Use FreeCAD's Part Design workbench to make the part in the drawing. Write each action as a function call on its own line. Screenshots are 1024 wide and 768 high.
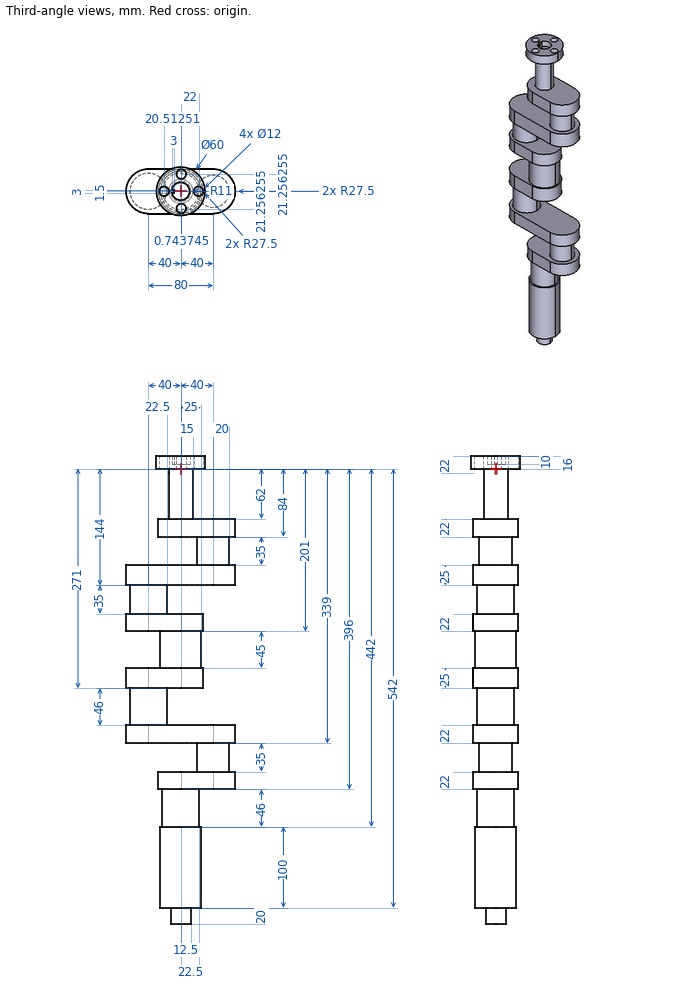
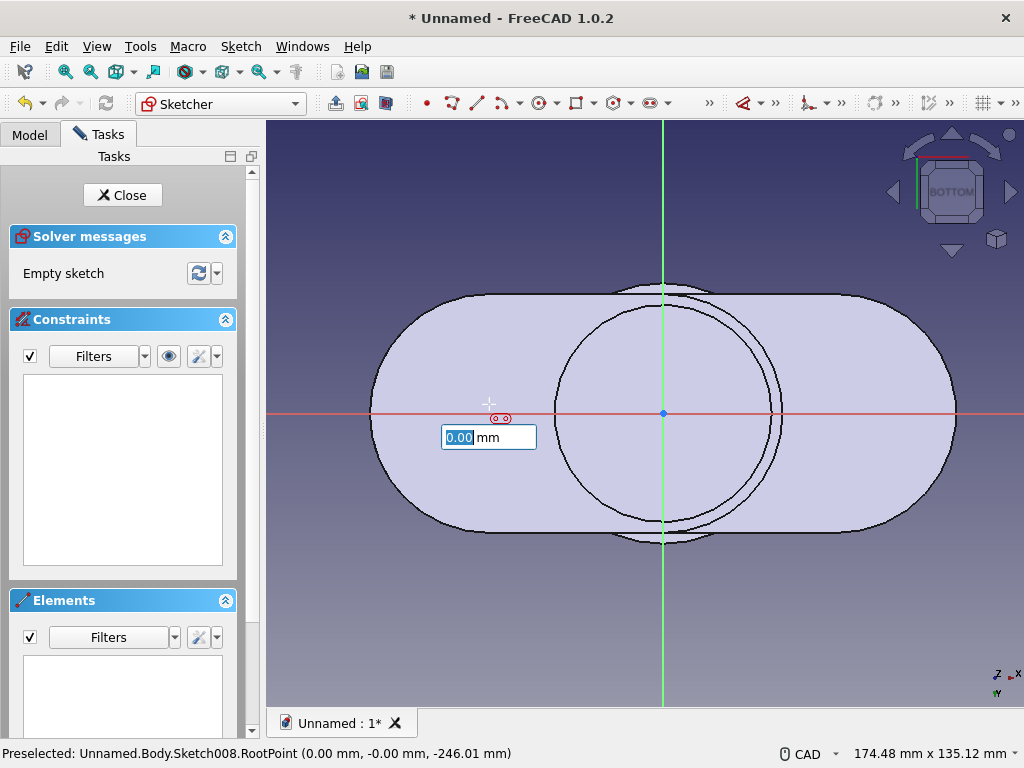
click(576, 533)
key(Escape)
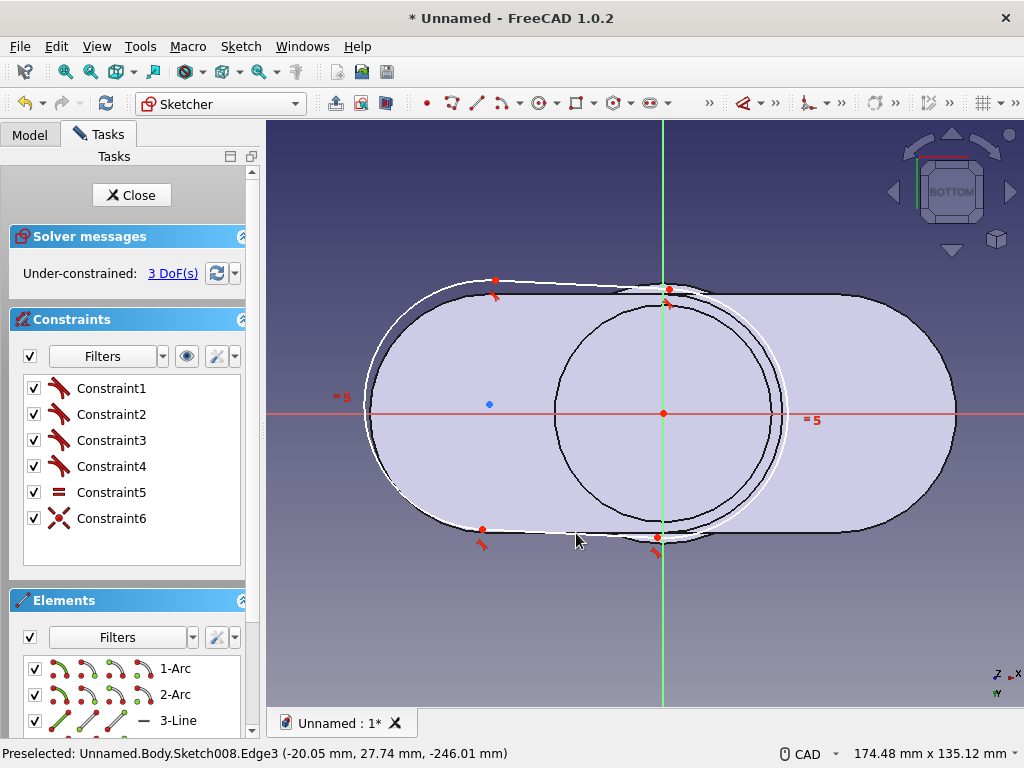
click(605, 535)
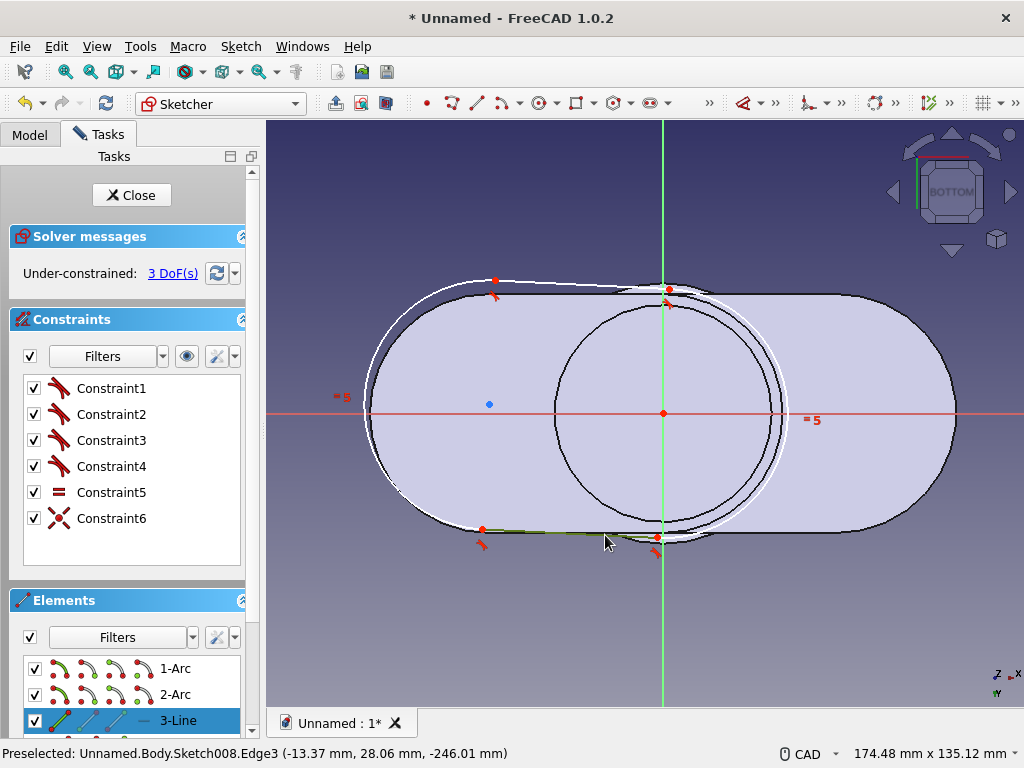
key(h)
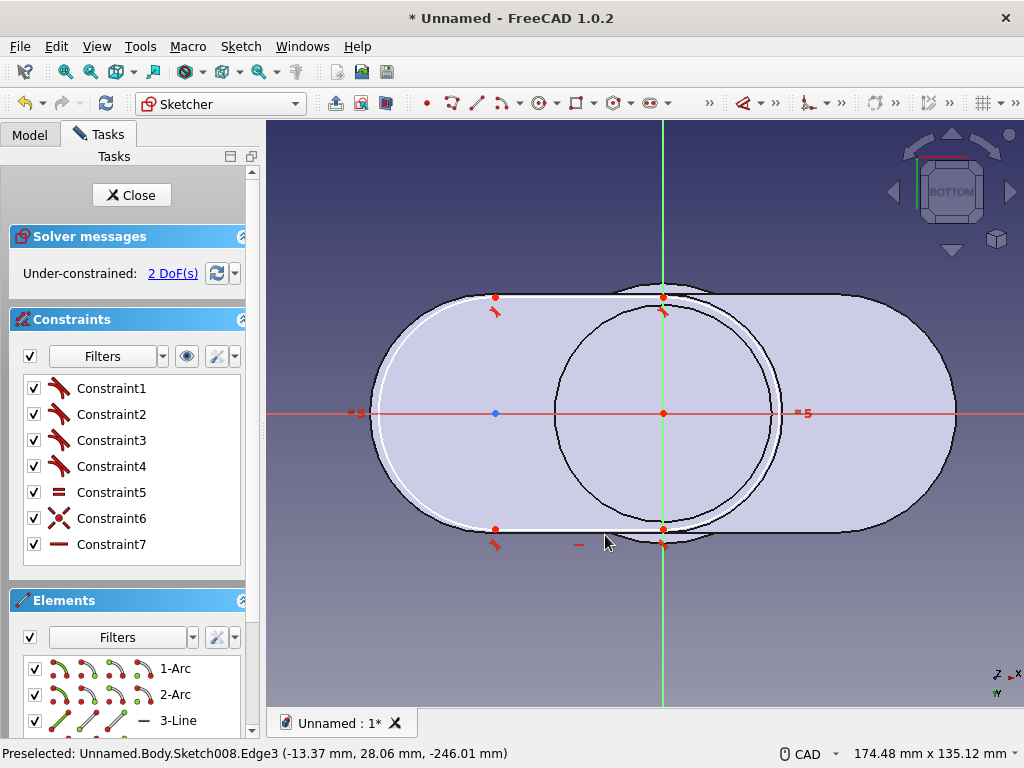
key(d)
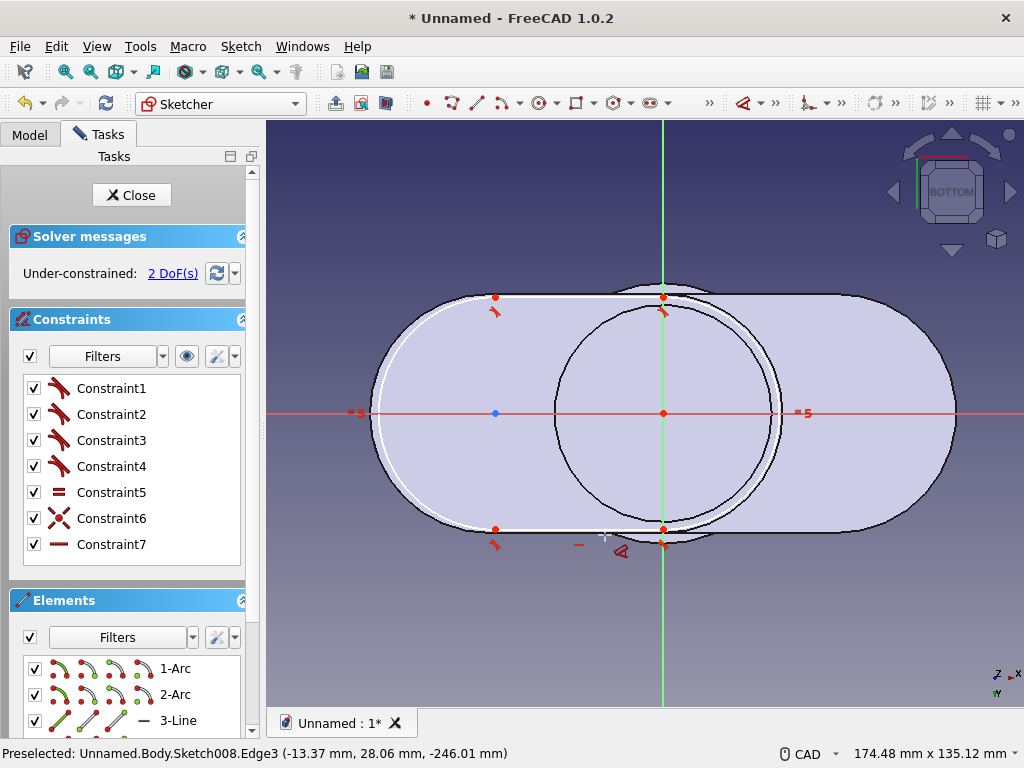
click(757, 482)
click(783, 501)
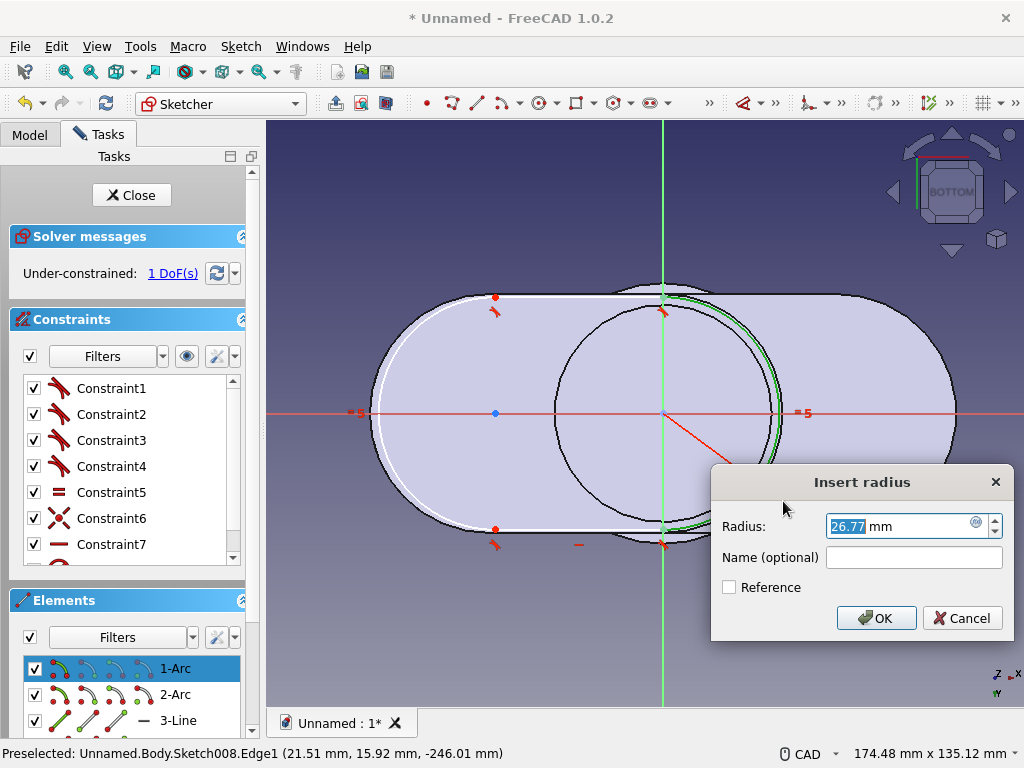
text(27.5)
key(Return)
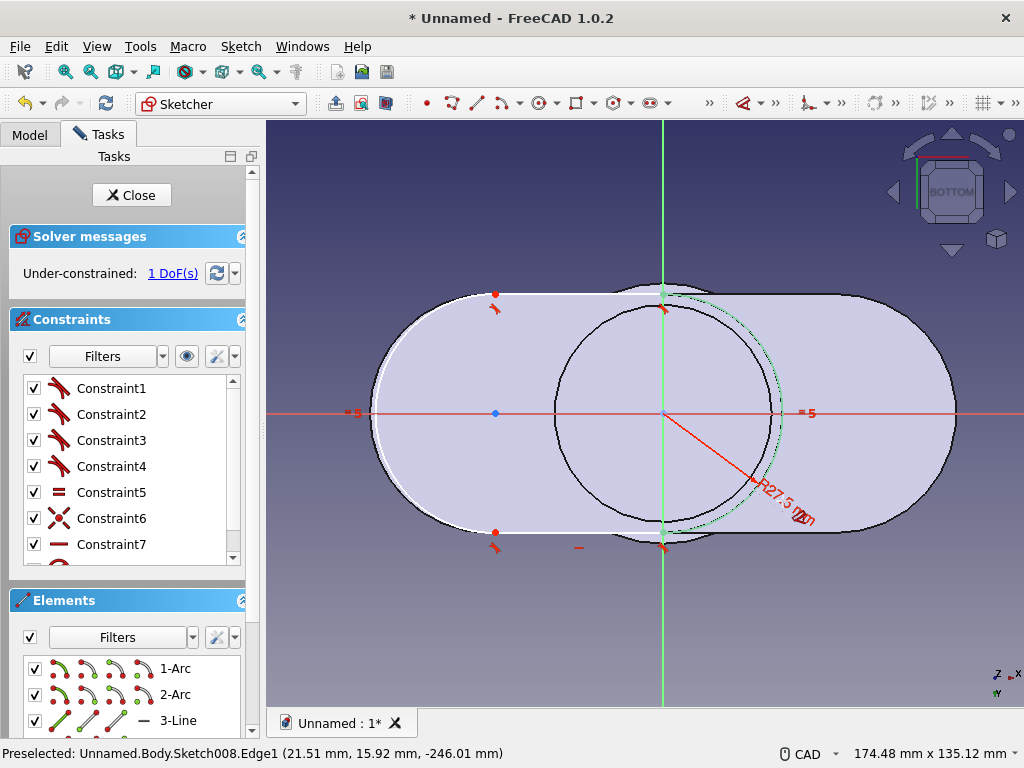
click(613, 533)
click(579, 567)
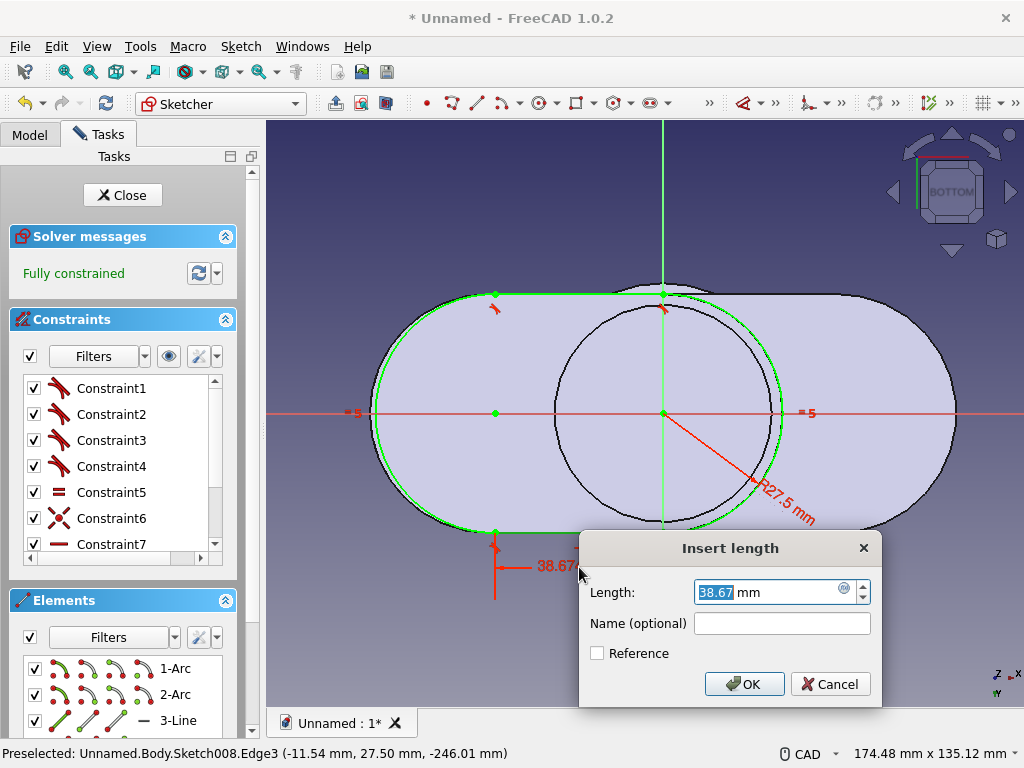
text(40)
key(Return)
key(Escape)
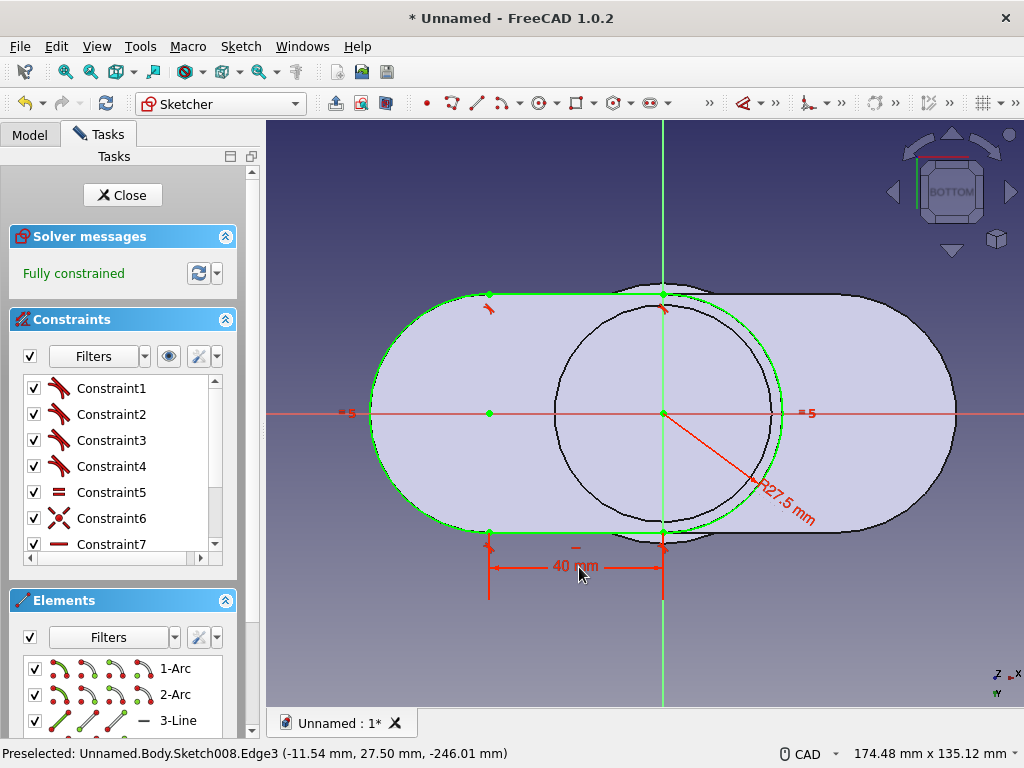
click(123, 195)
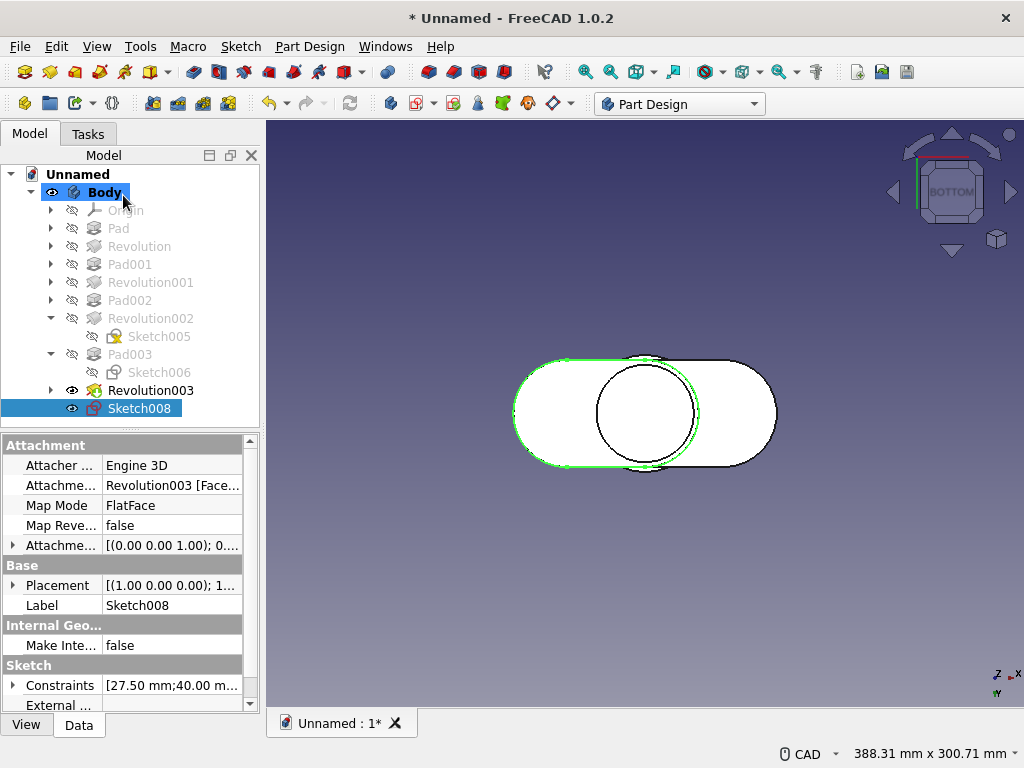
click(25, 72)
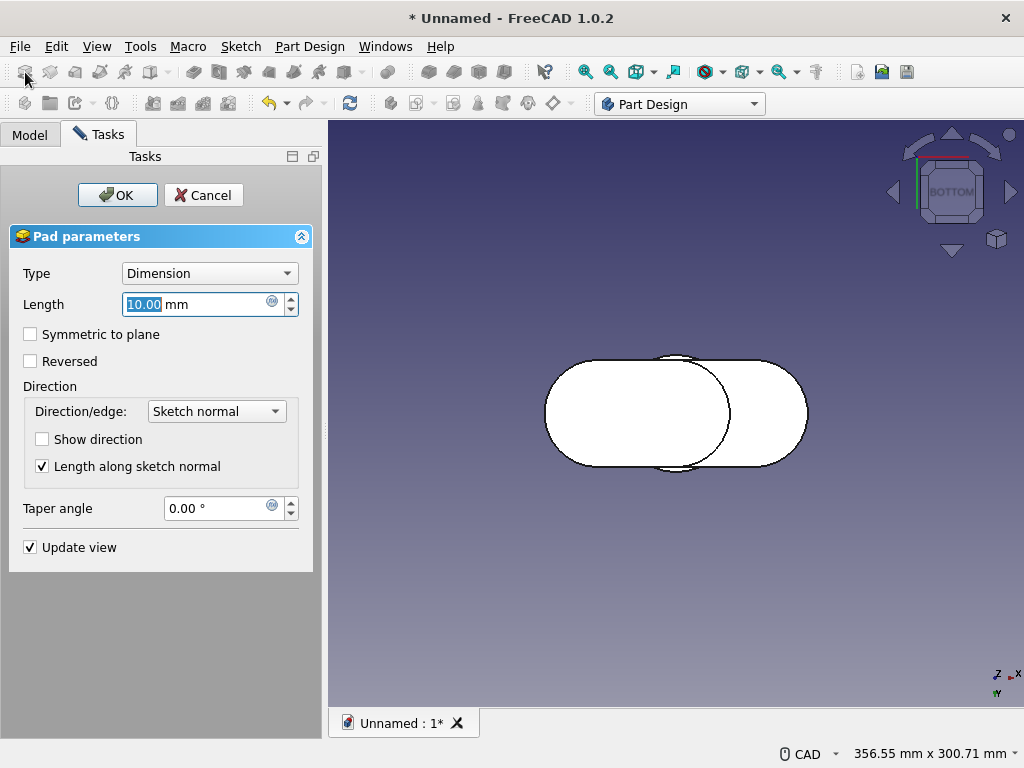
text(25)
key(Tab)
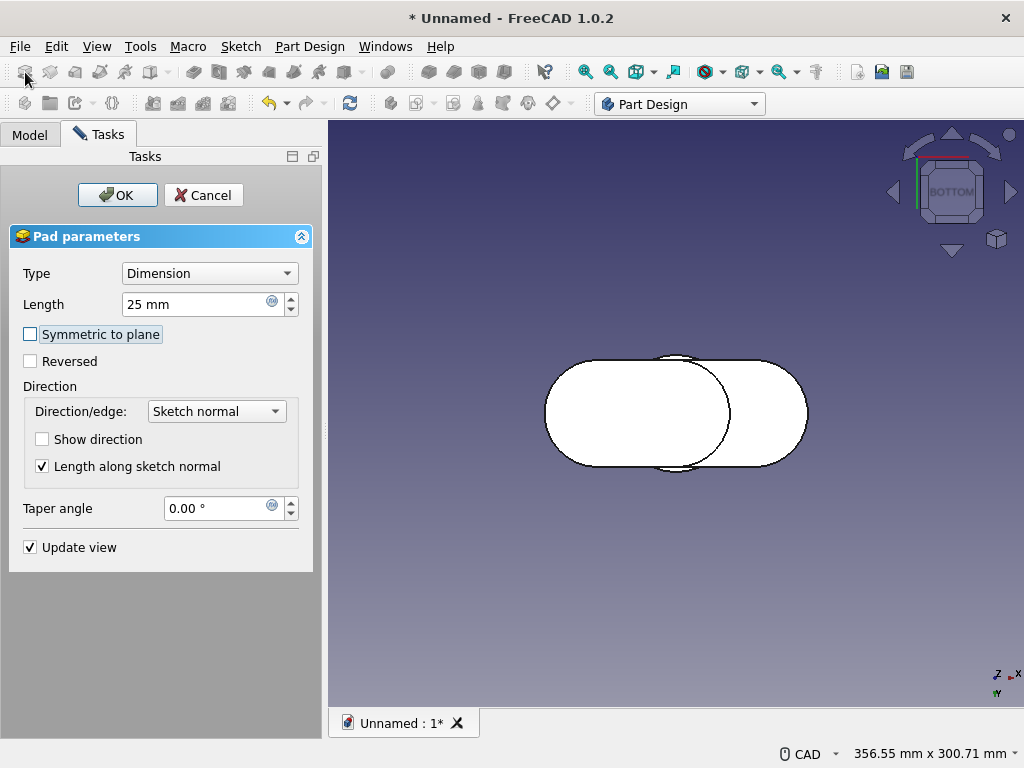
click(118, 195)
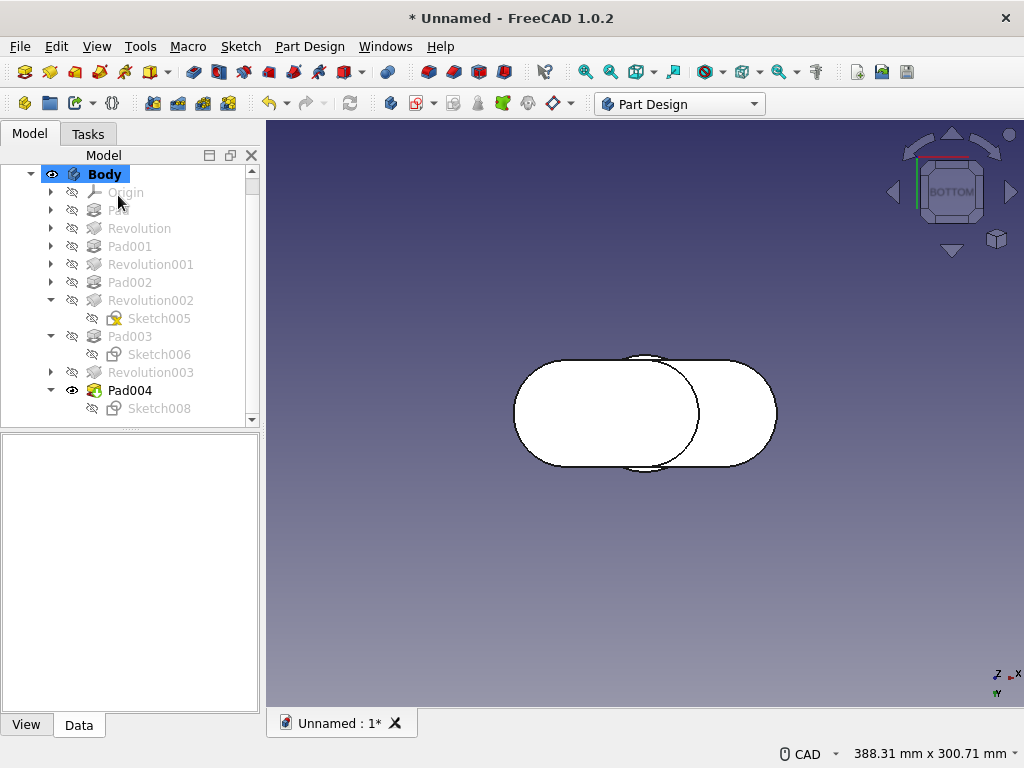
key(v)
key(f)